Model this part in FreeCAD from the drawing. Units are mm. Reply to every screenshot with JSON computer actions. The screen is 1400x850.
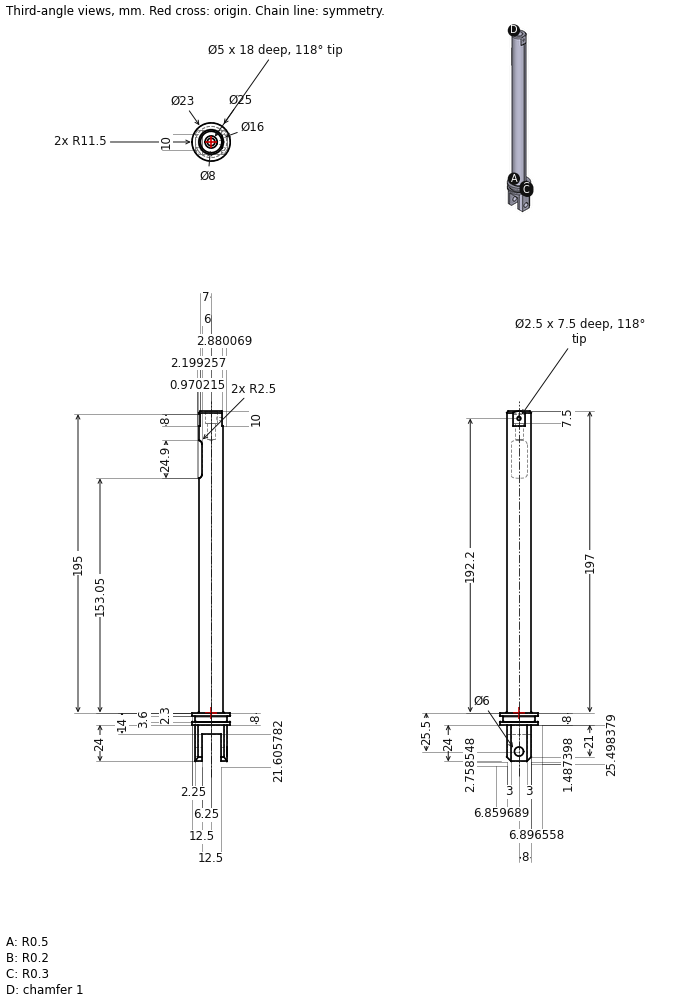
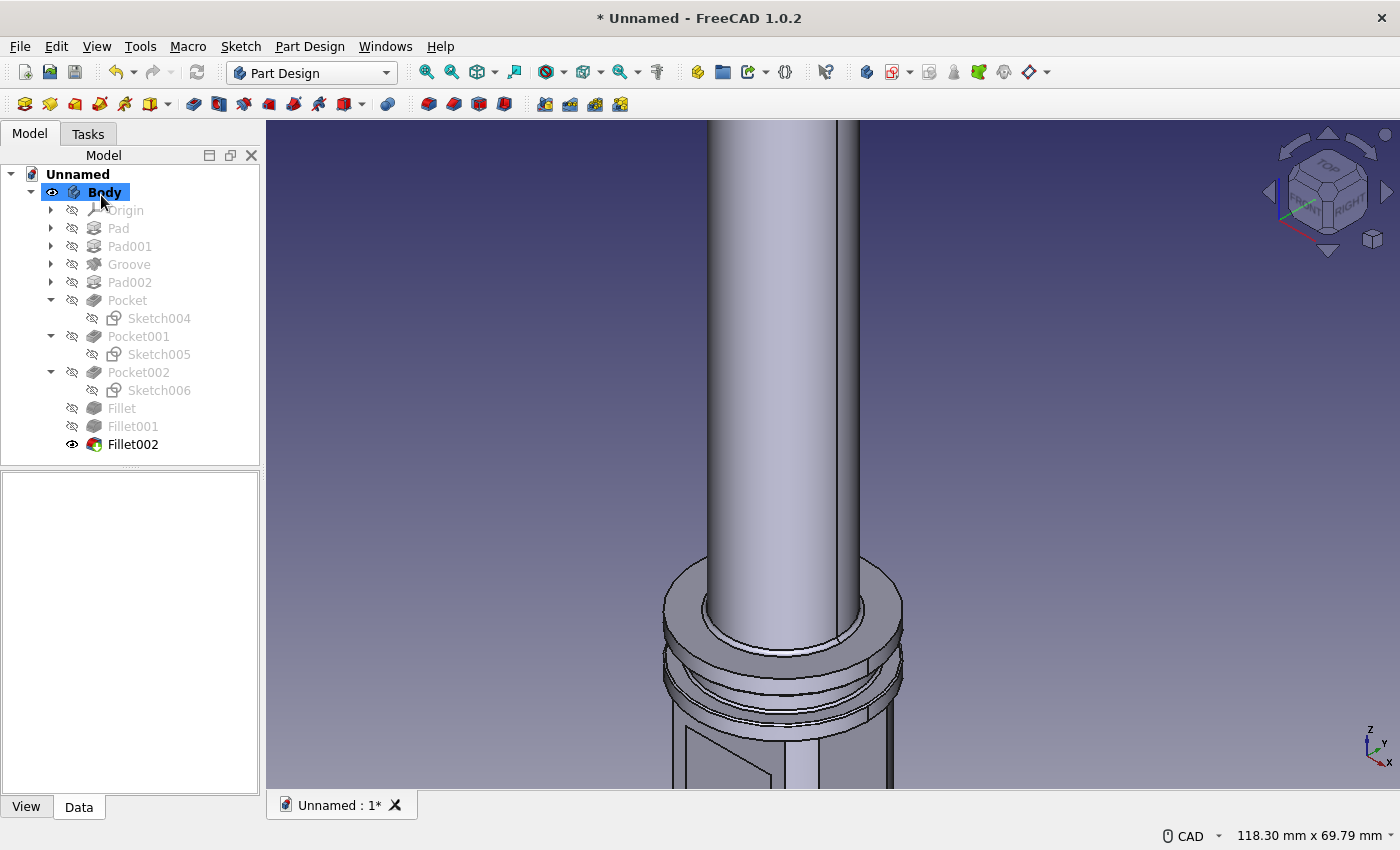
{"action": "left_click", "coordinate": [427, 72]}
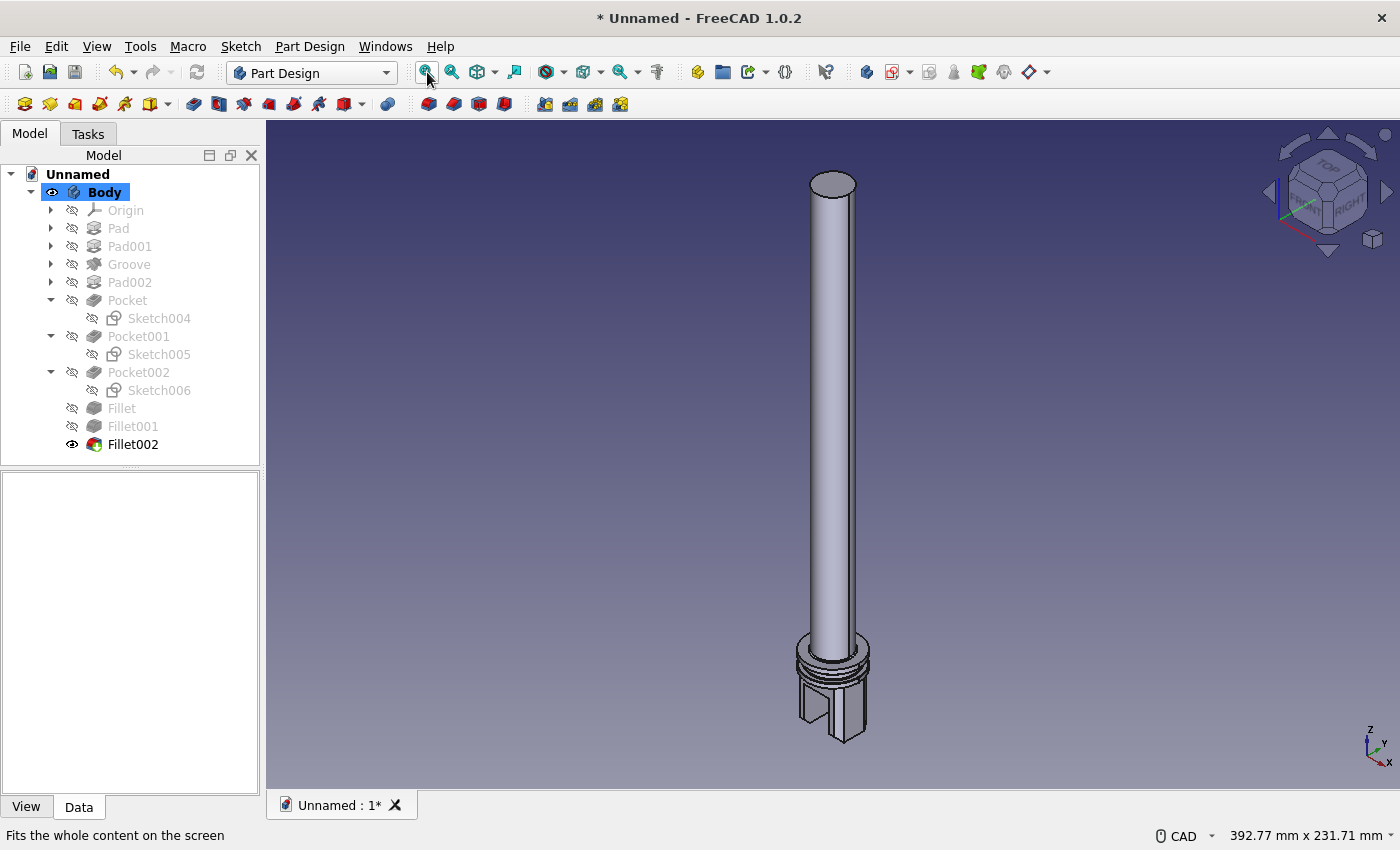
{"action": "left_click", "coordinate": [810, 181]}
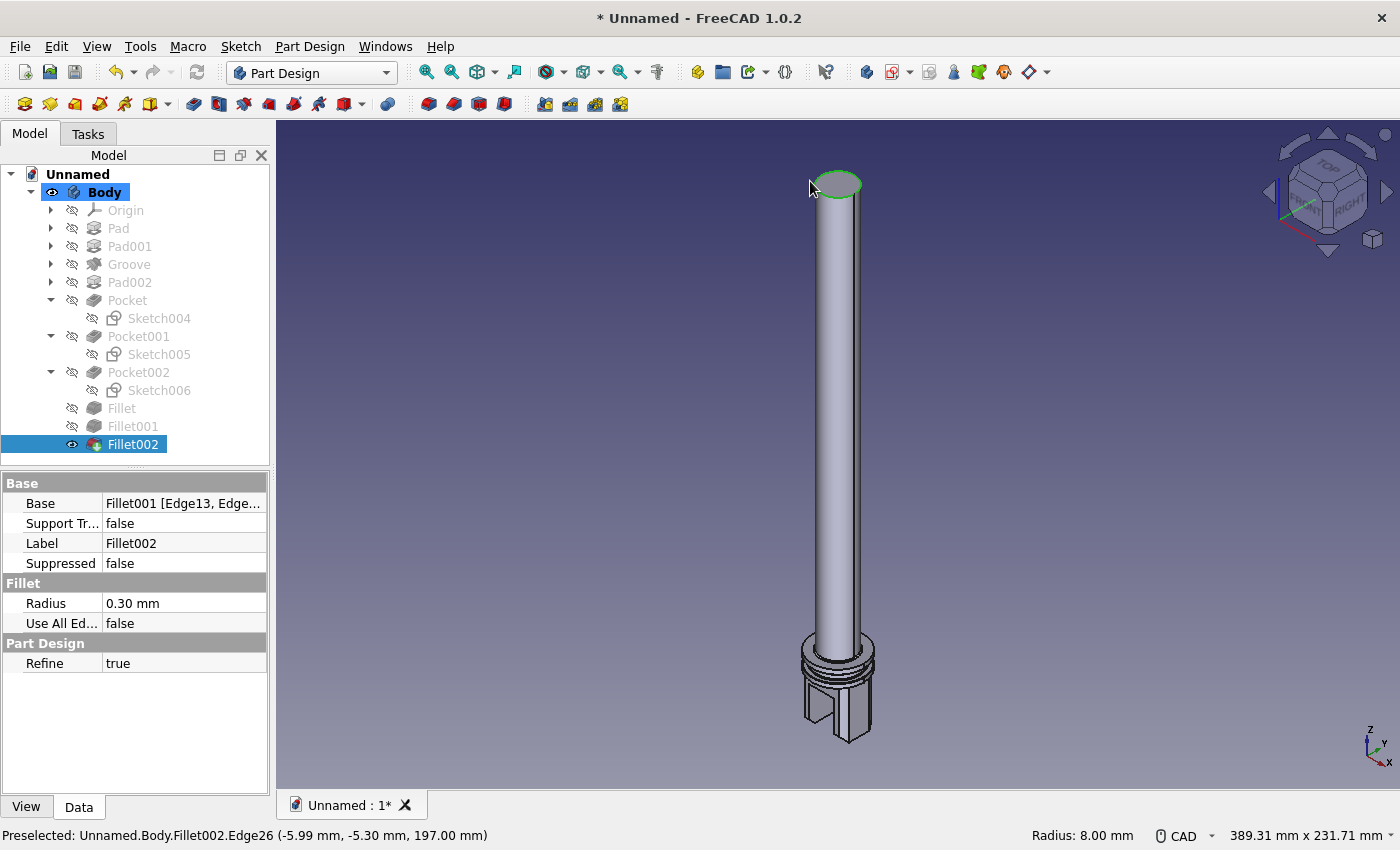
{"action": "left_click", "coordinate": [454, 104]}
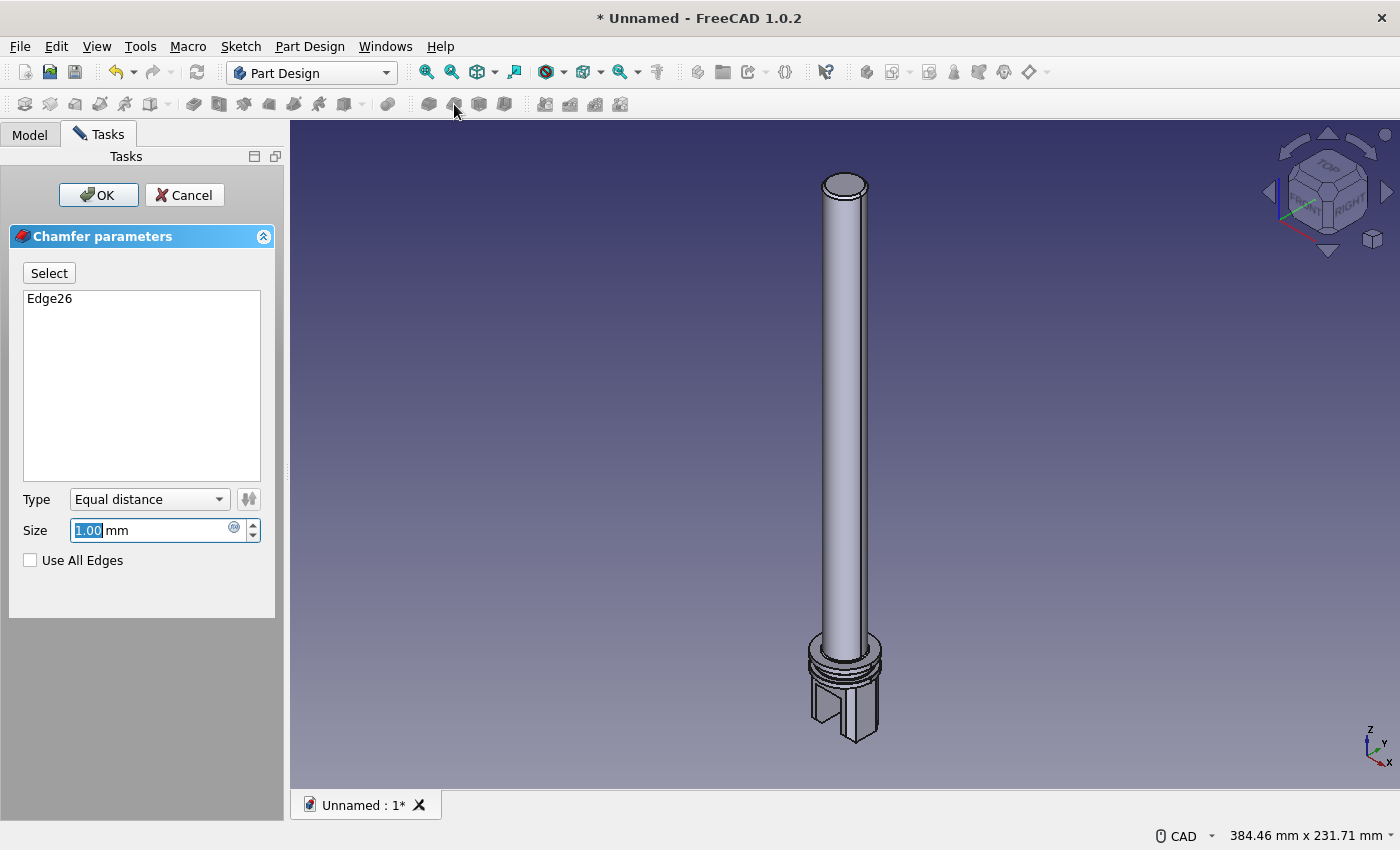
{"action": "type", "text": "1"}
{"action": "key", "text": "Tab"}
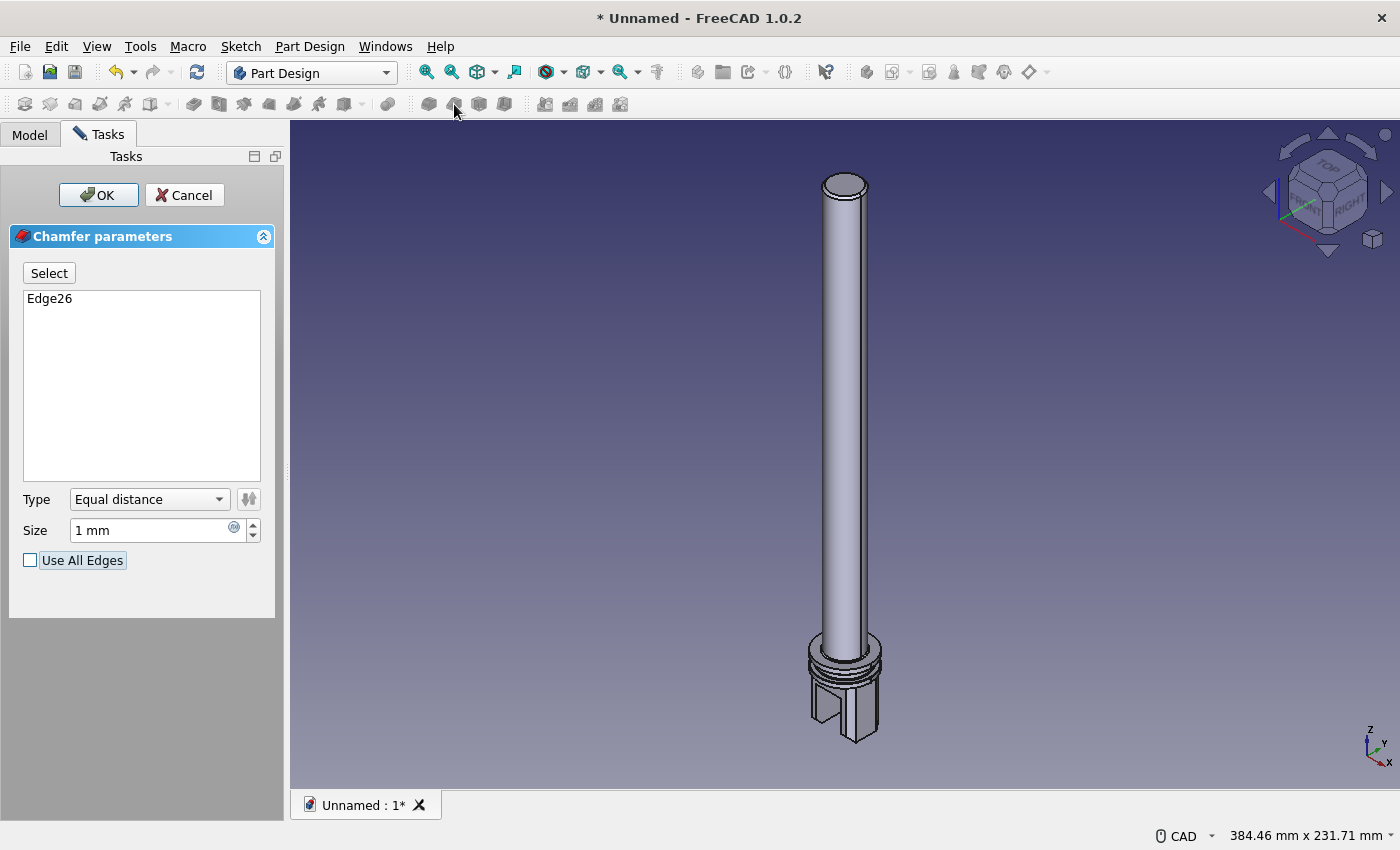
{"action": "left_click", "coordinate": [99, 195]}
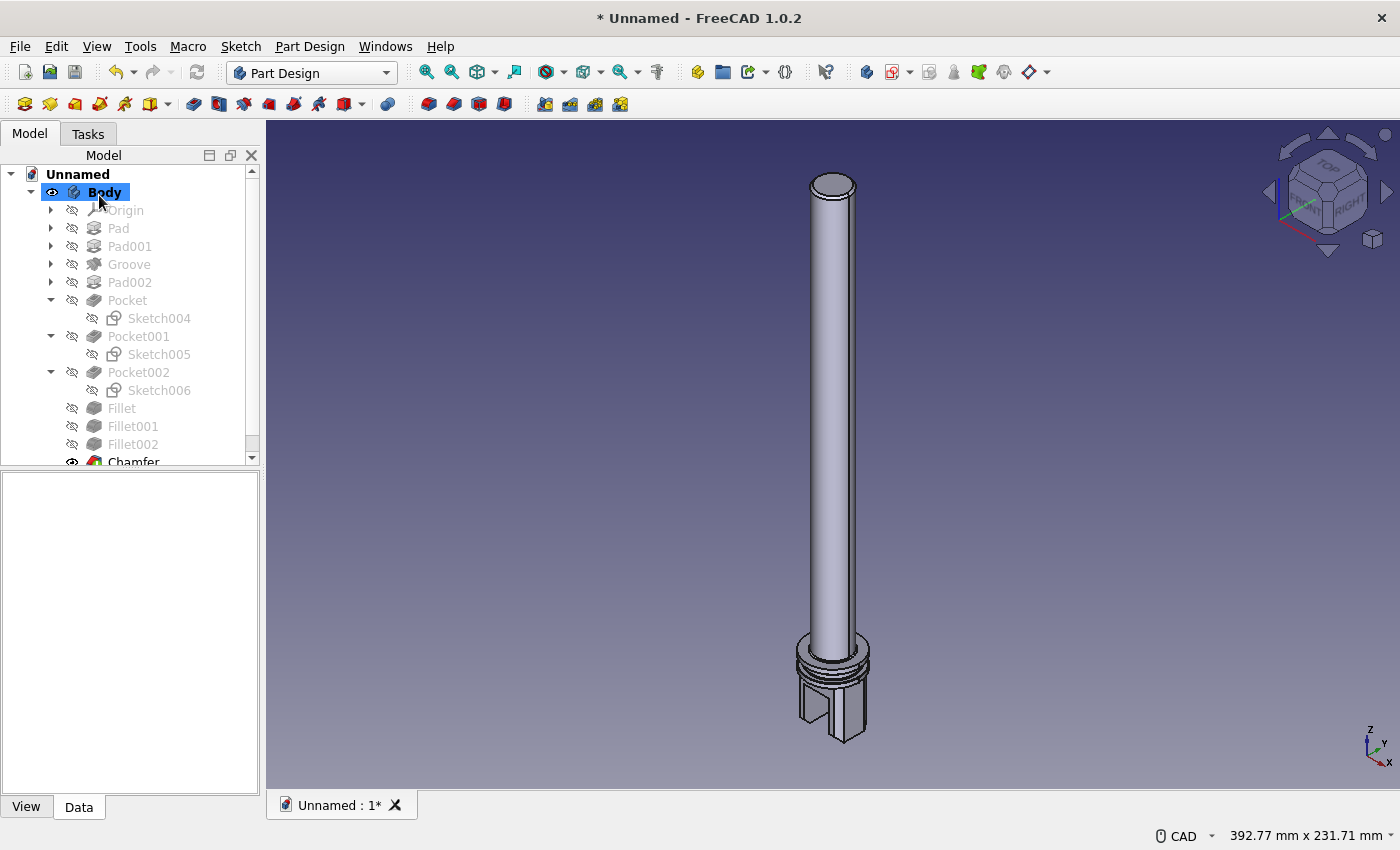
{"action": "key", "text": "4"}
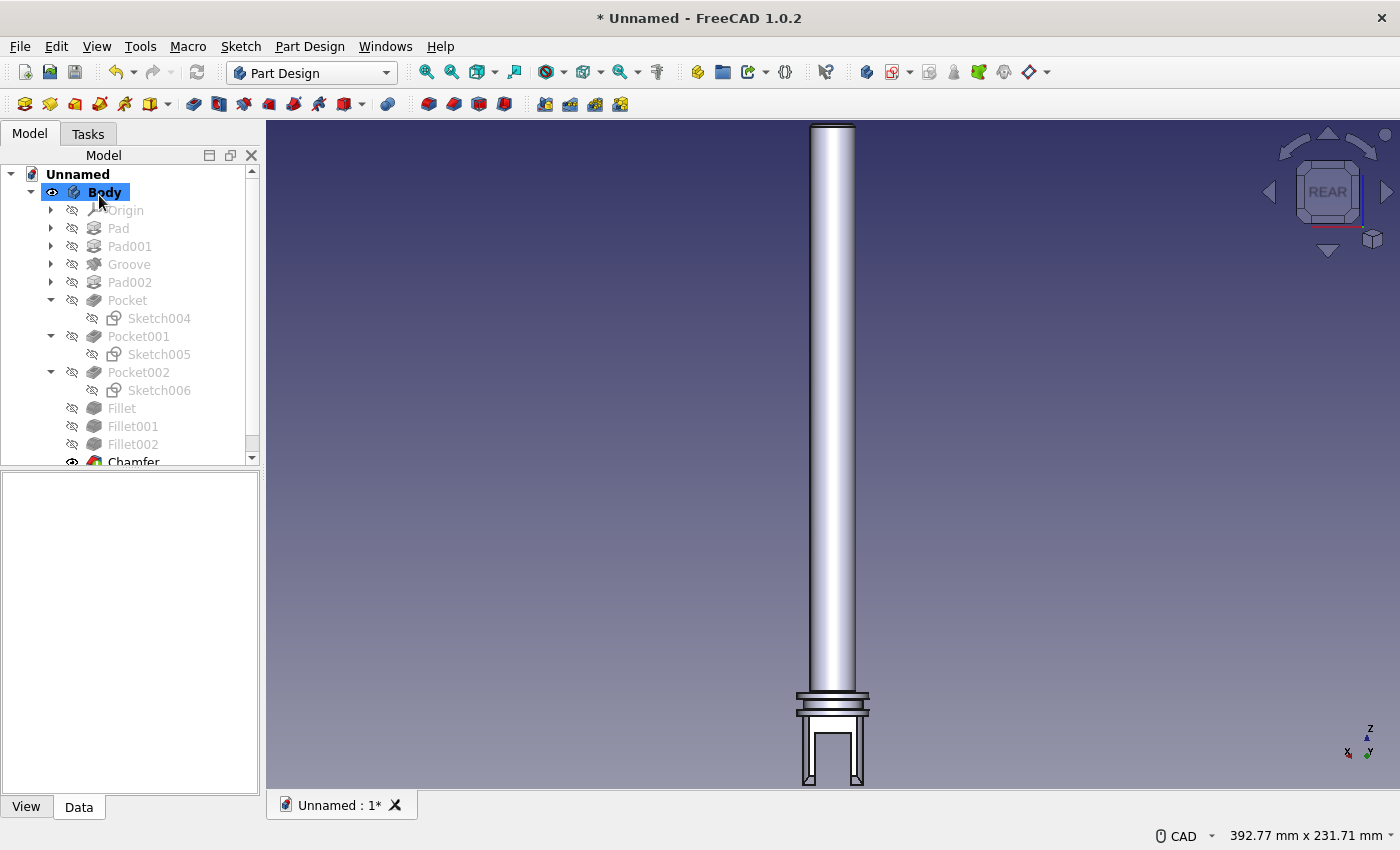
{"action": "scroll", "coordinate": [819, 719], "scroll_direction": "up", "scroll_amount": 6}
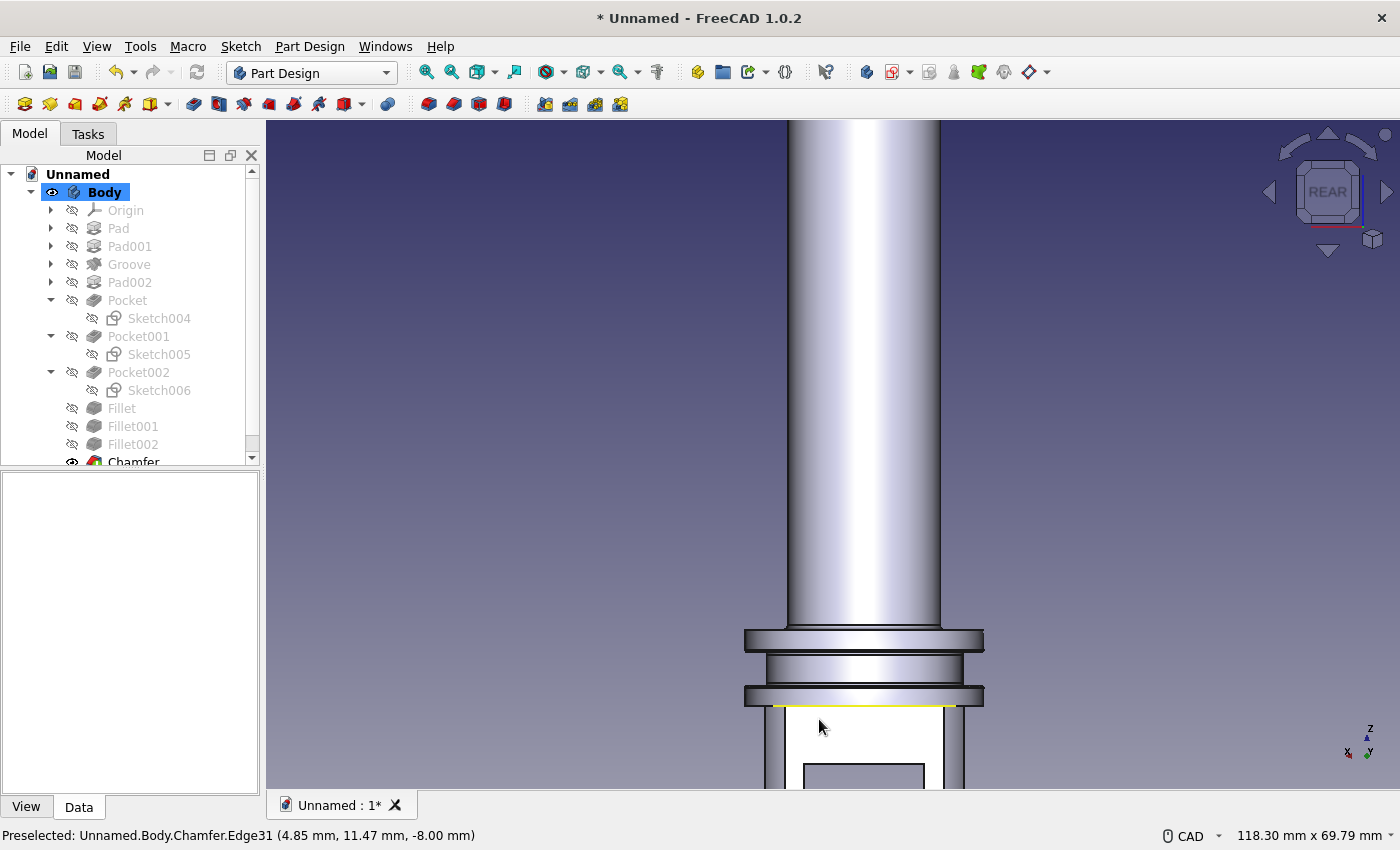
{"action": "left_click", "coordinate": [819, 720]}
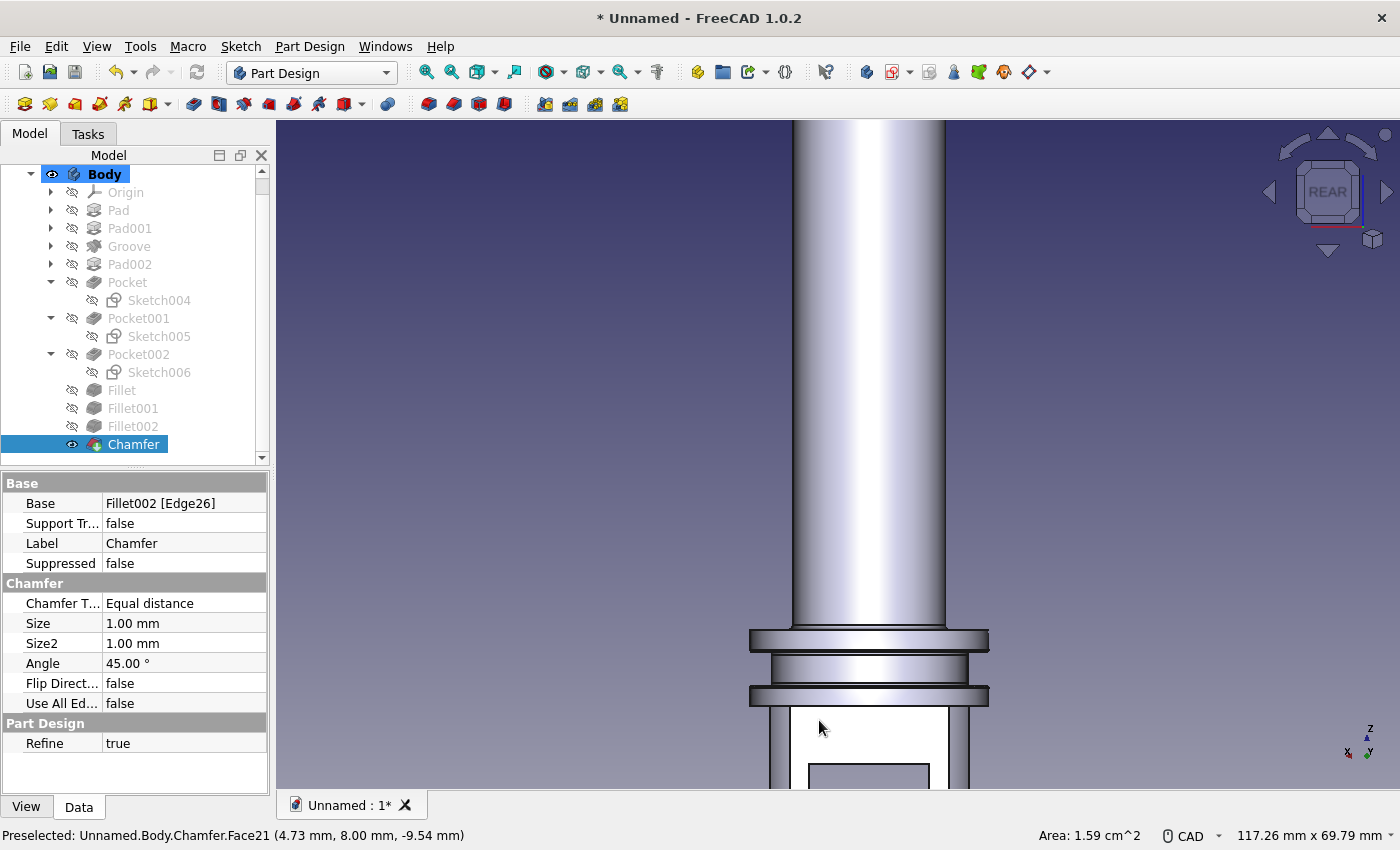
{"action": "left_click", "coordinate": [892, 72]}